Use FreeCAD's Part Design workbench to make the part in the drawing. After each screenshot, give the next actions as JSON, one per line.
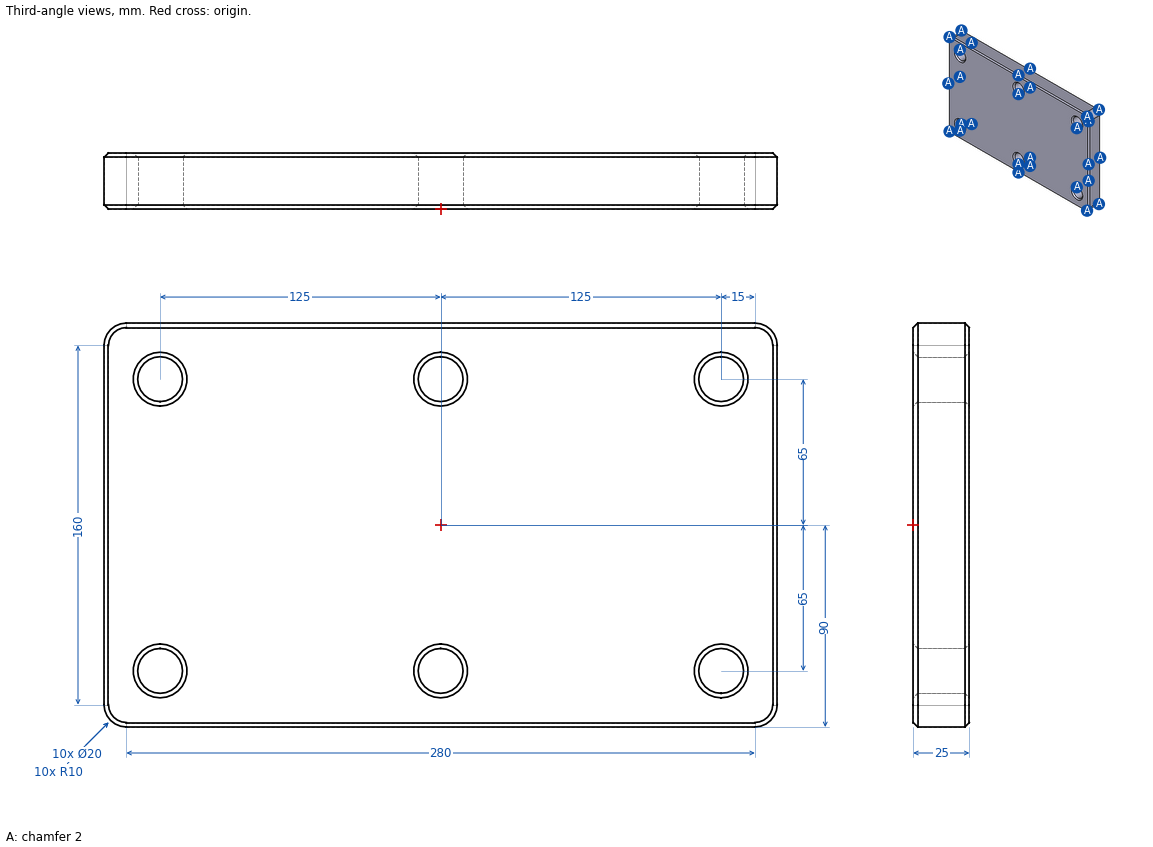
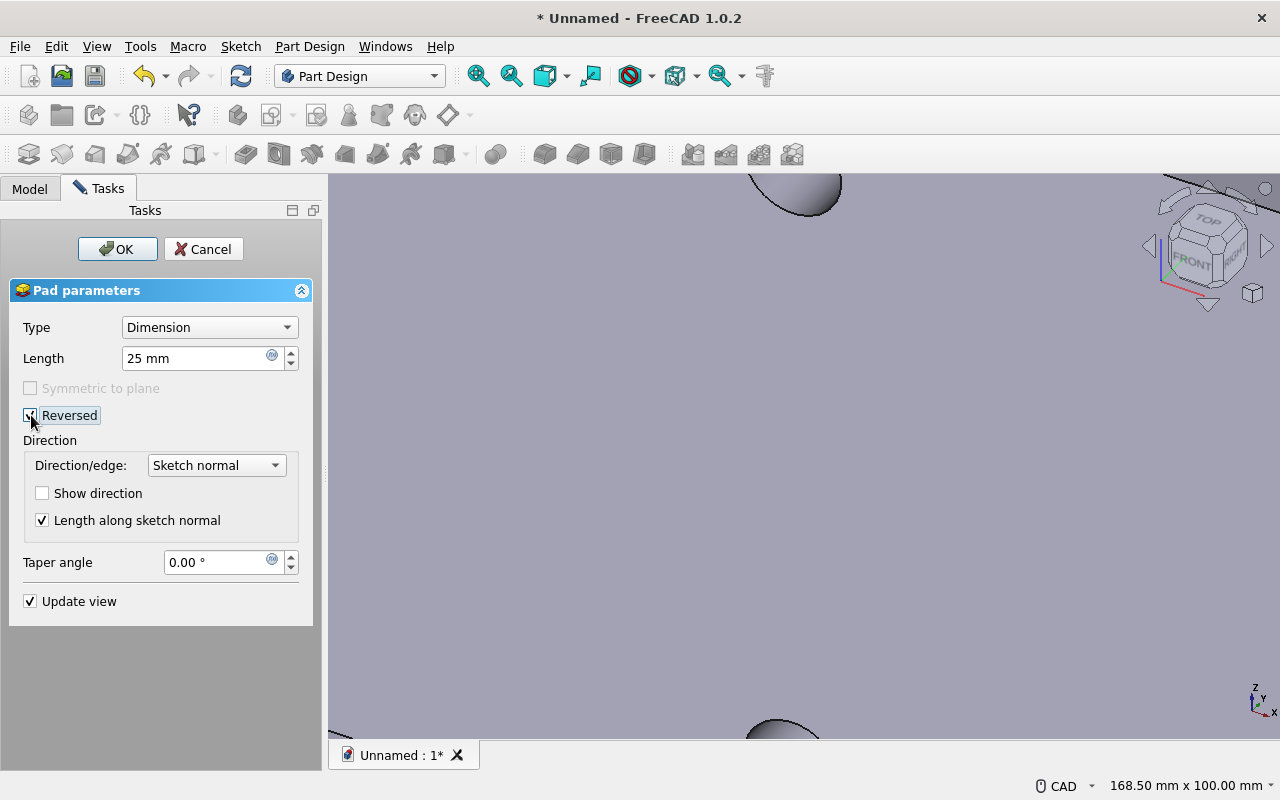
{"action": "left_click", "coordinate": [118, 249]}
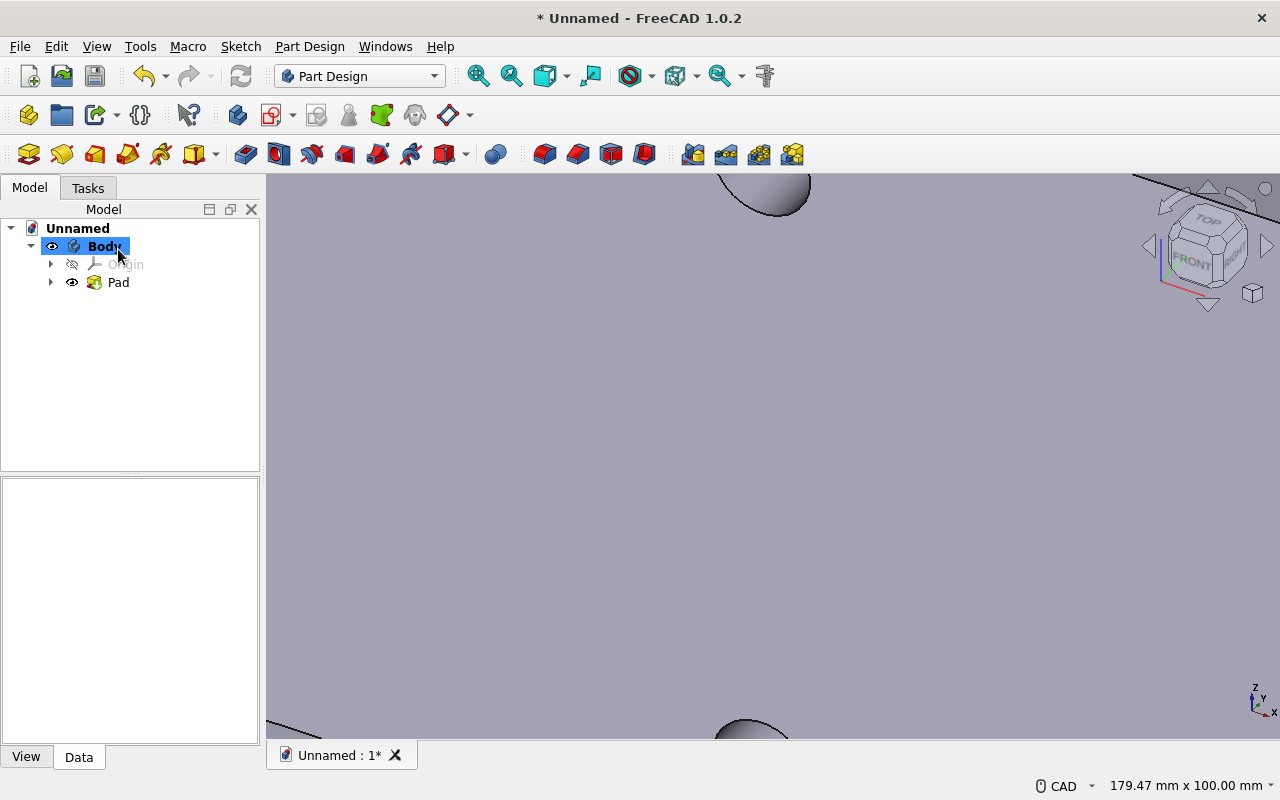
{"action": "left_click", "coordinate": [479, 76]}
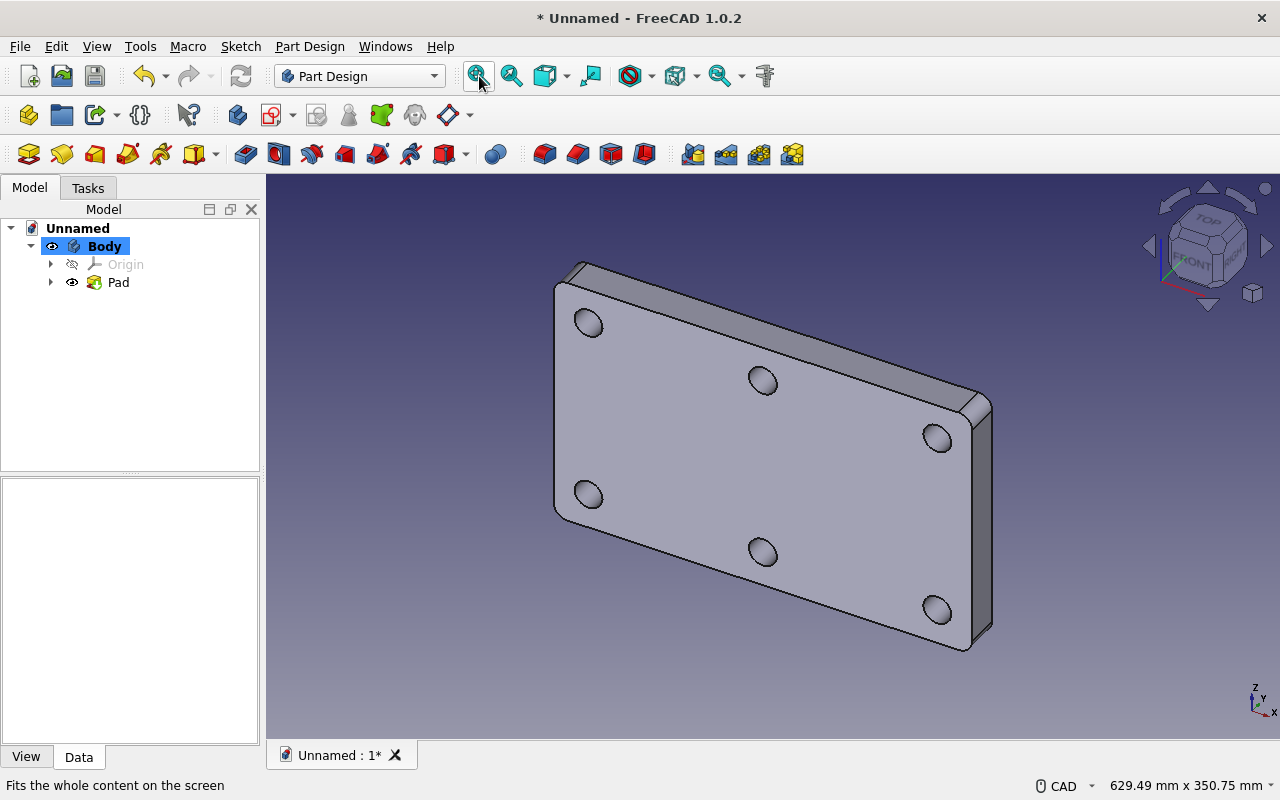
{"action": "left_click", "coordinate": [703, 446]}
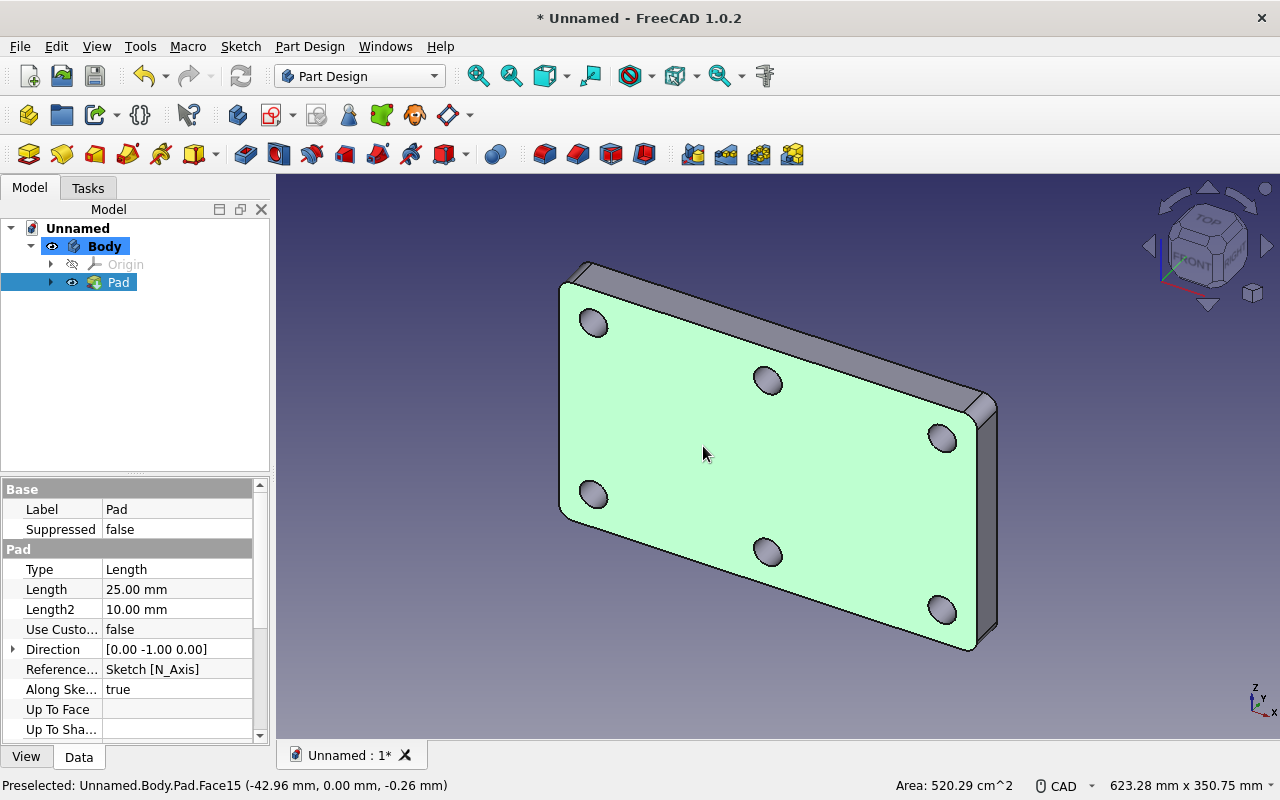
{"action": "key", "text": "0"}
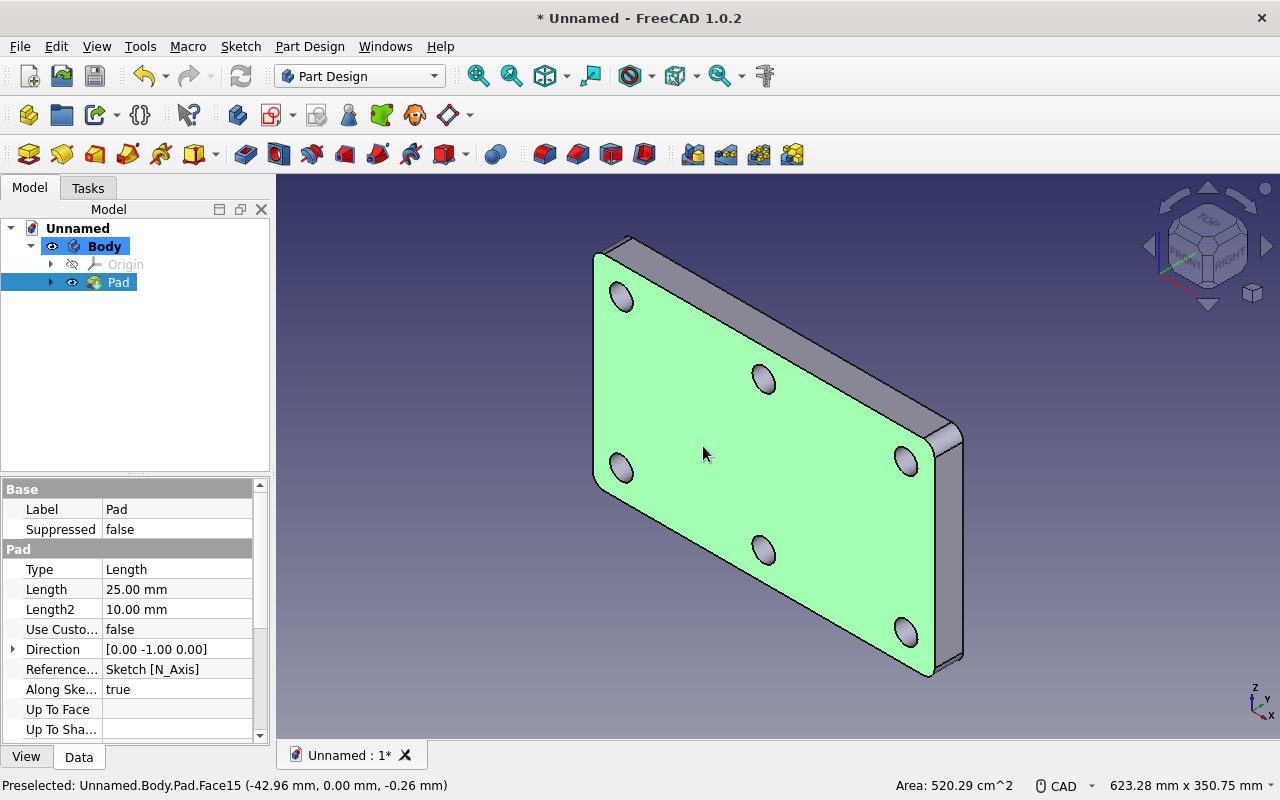
{"action": "key", "text": "2"}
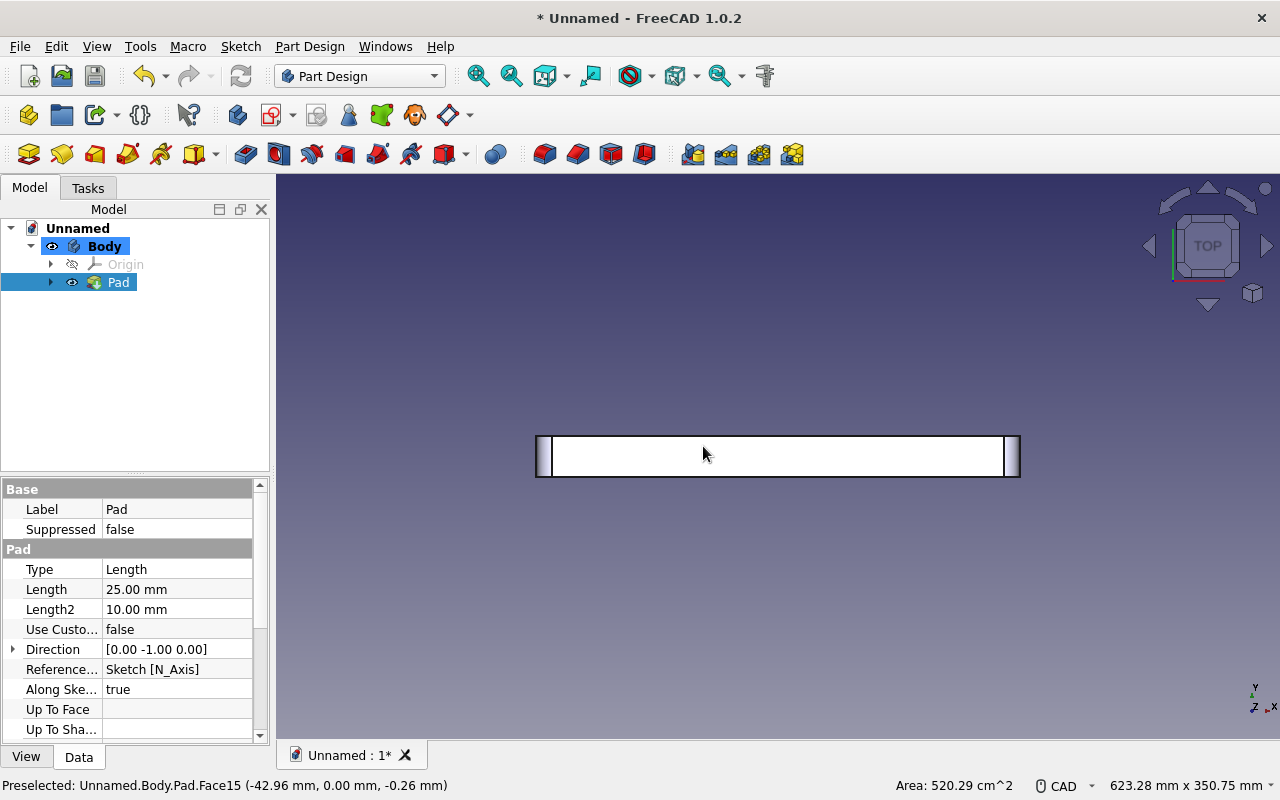
{"action": "key", "text": "1"}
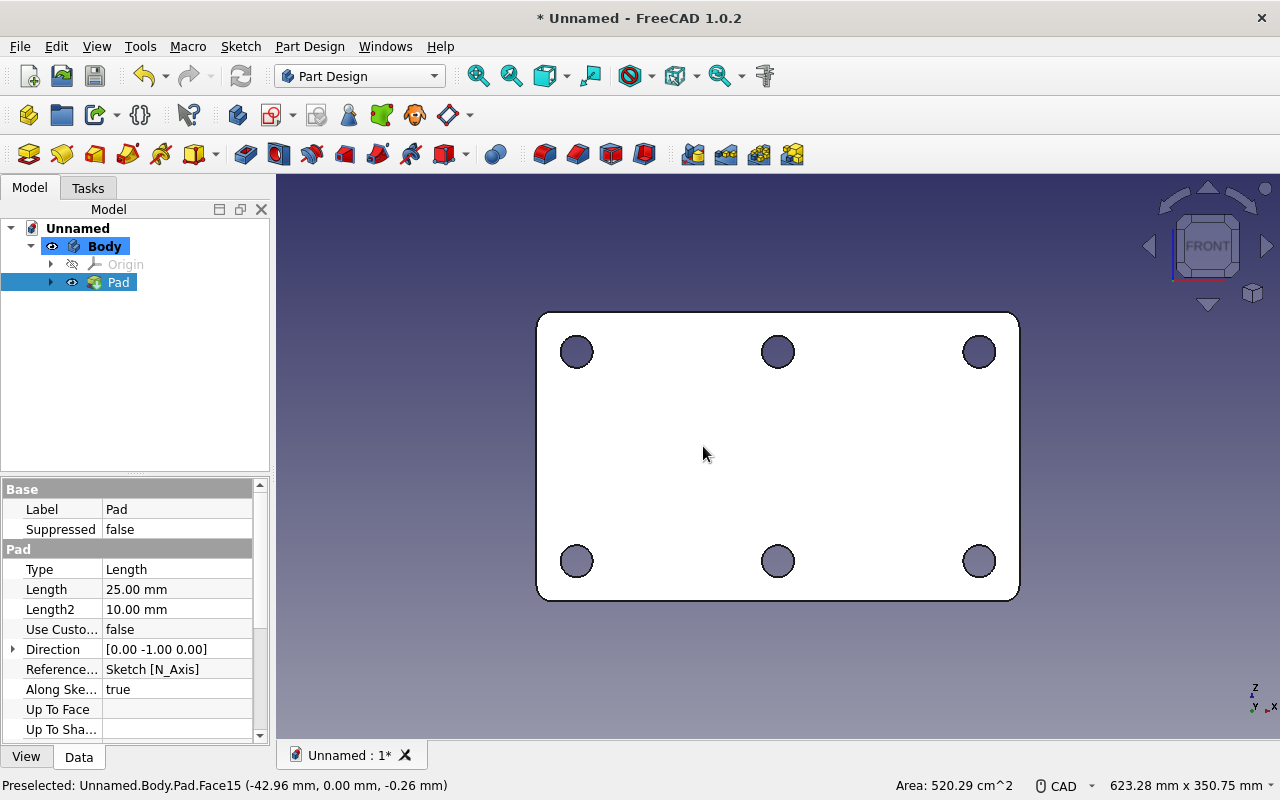
{"action": "key", "text": "3"}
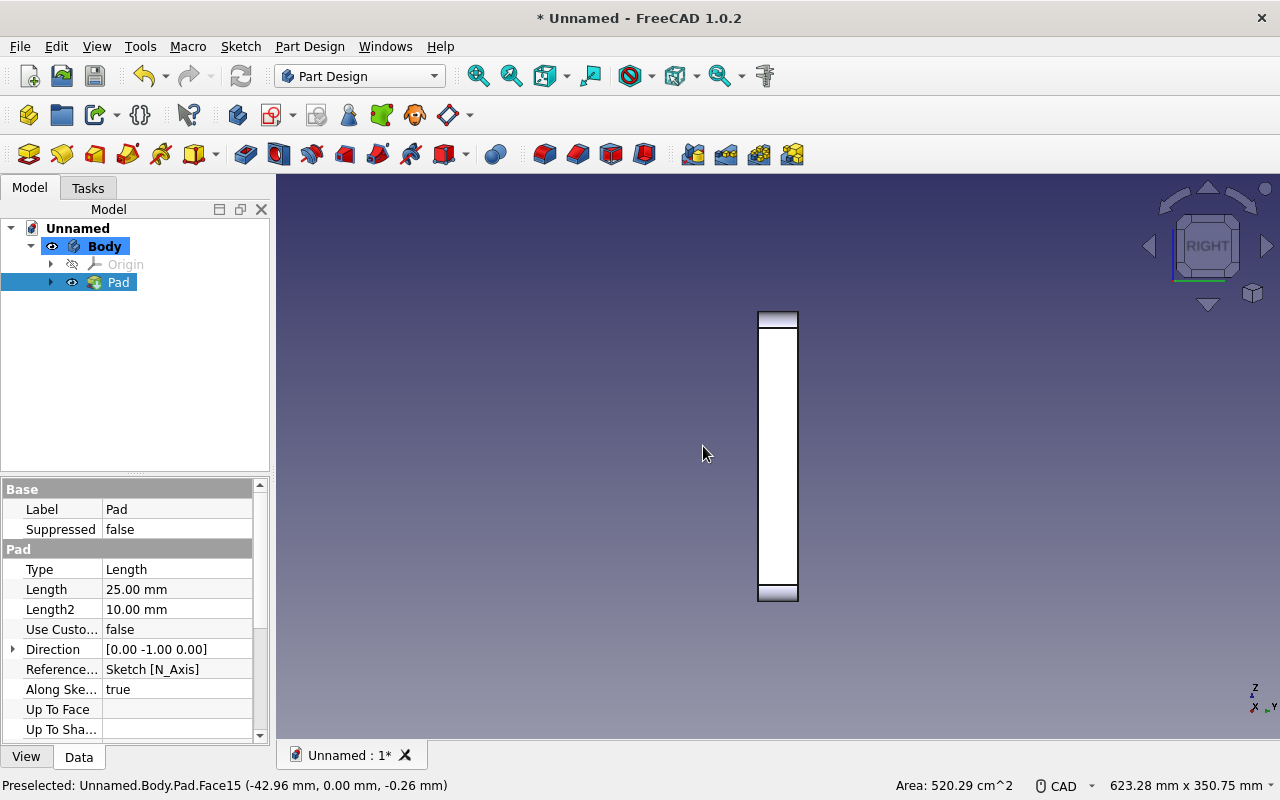
{"action": "key", "text": "5"}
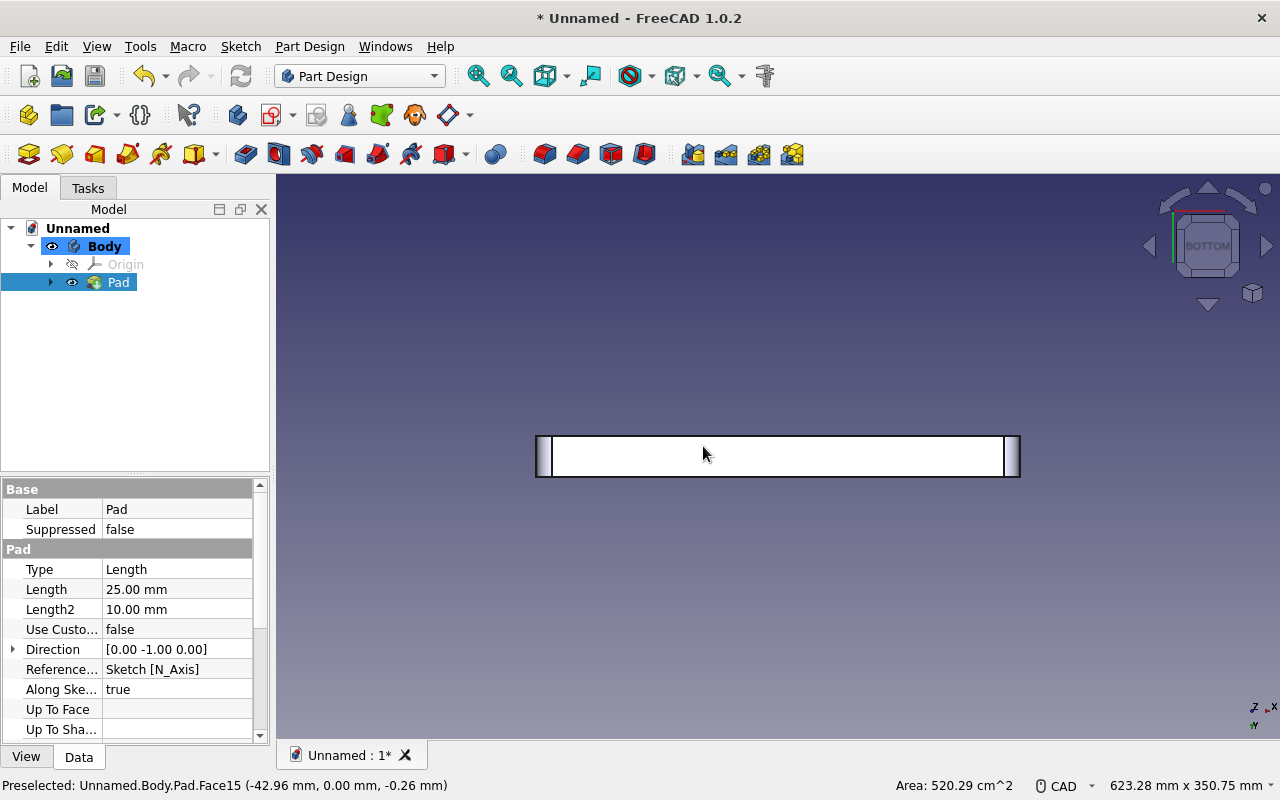
{"action": "key", "text": "4"}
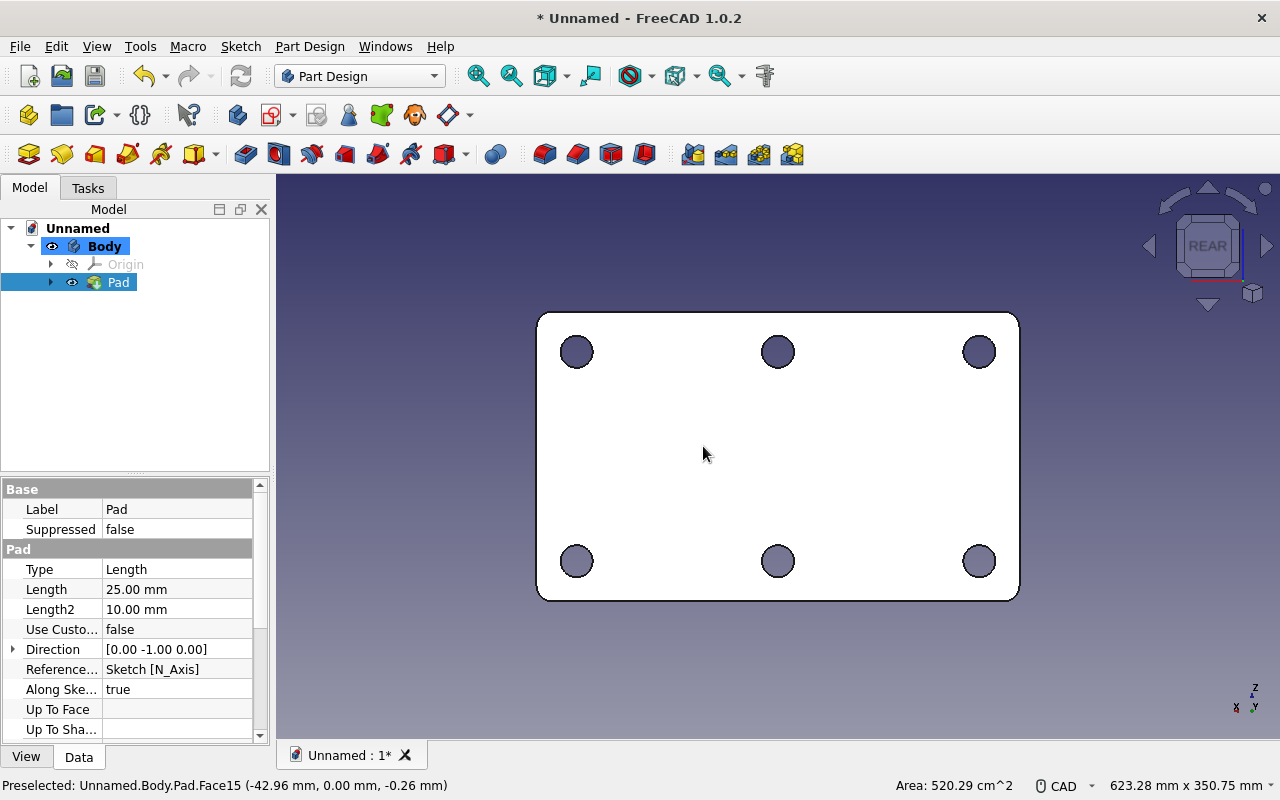
{"action": "left_click", "coordinate": [847, 456], "text": "ctrl"}